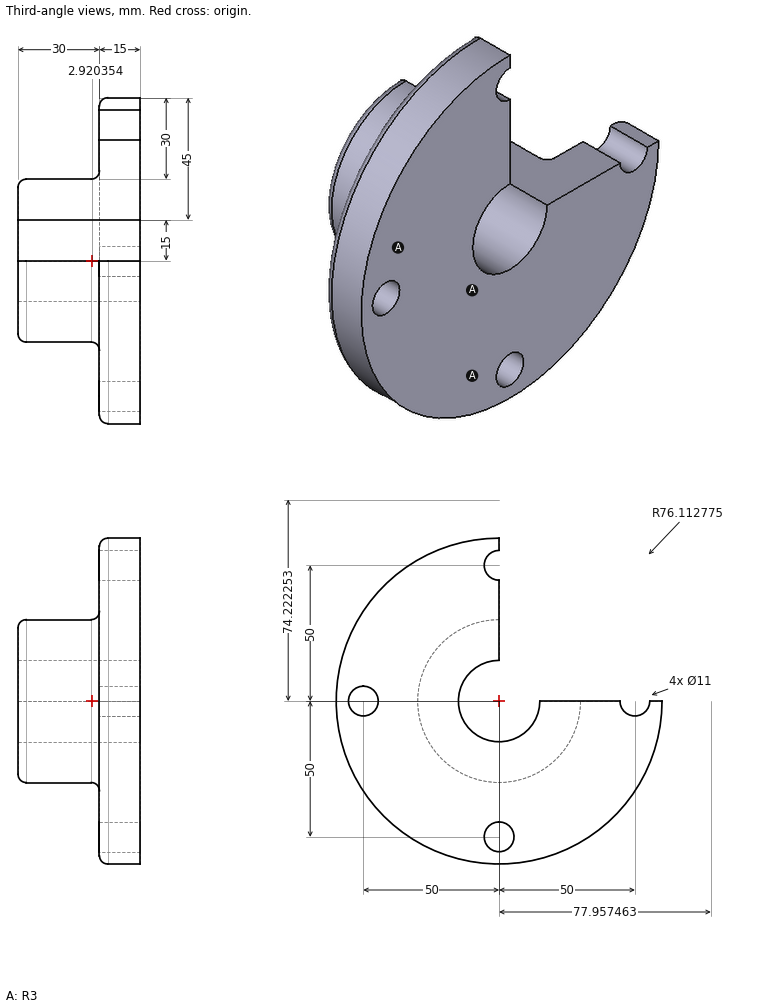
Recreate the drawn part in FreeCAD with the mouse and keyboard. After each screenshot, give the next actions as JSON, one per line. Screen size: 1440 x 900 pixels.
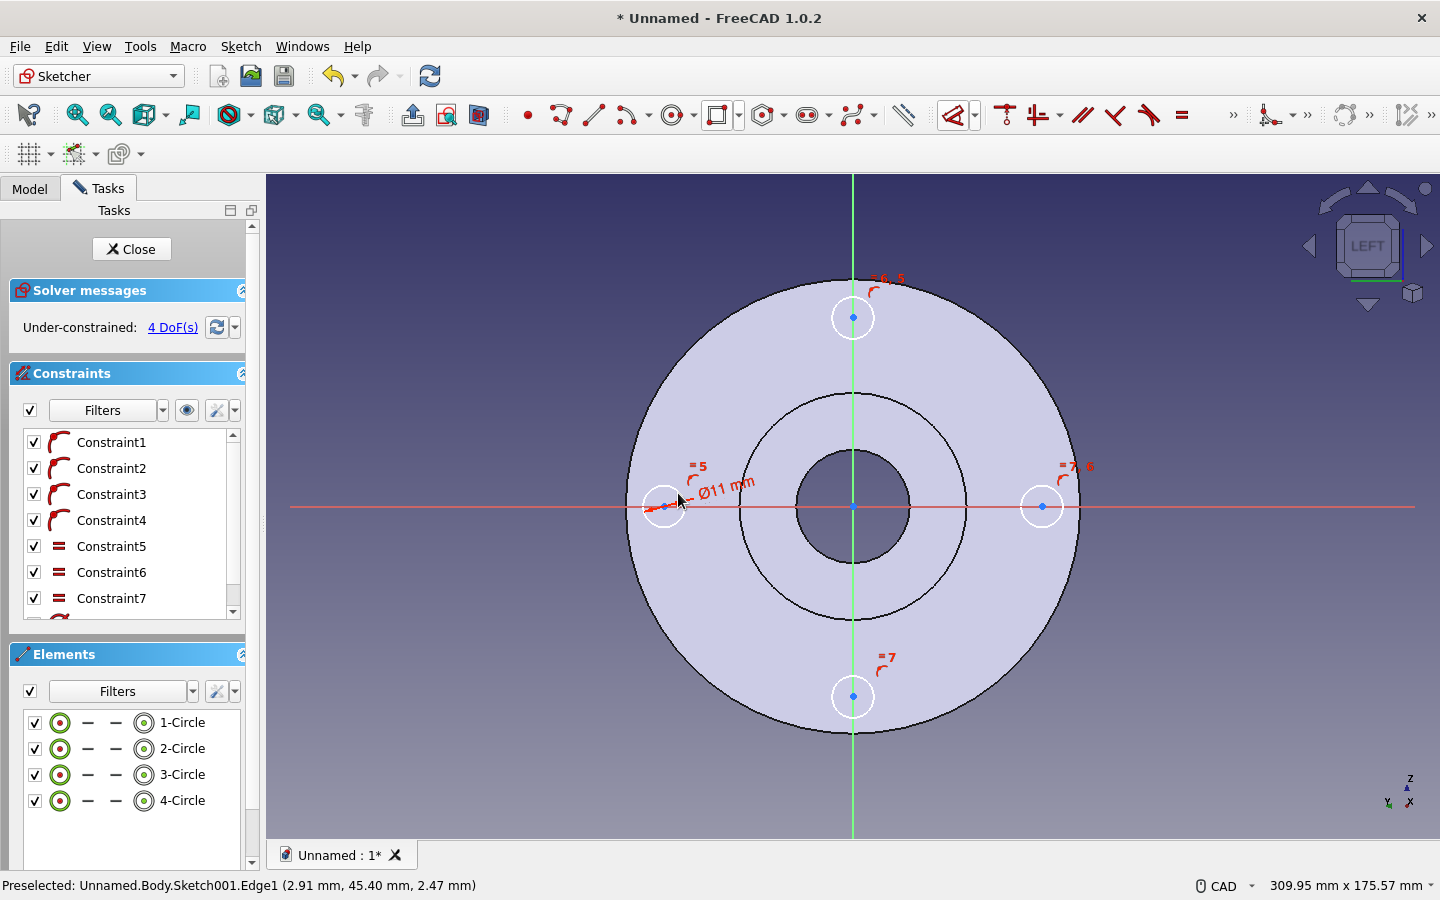
{"action": "left_click", "coordinate": [664, 506]}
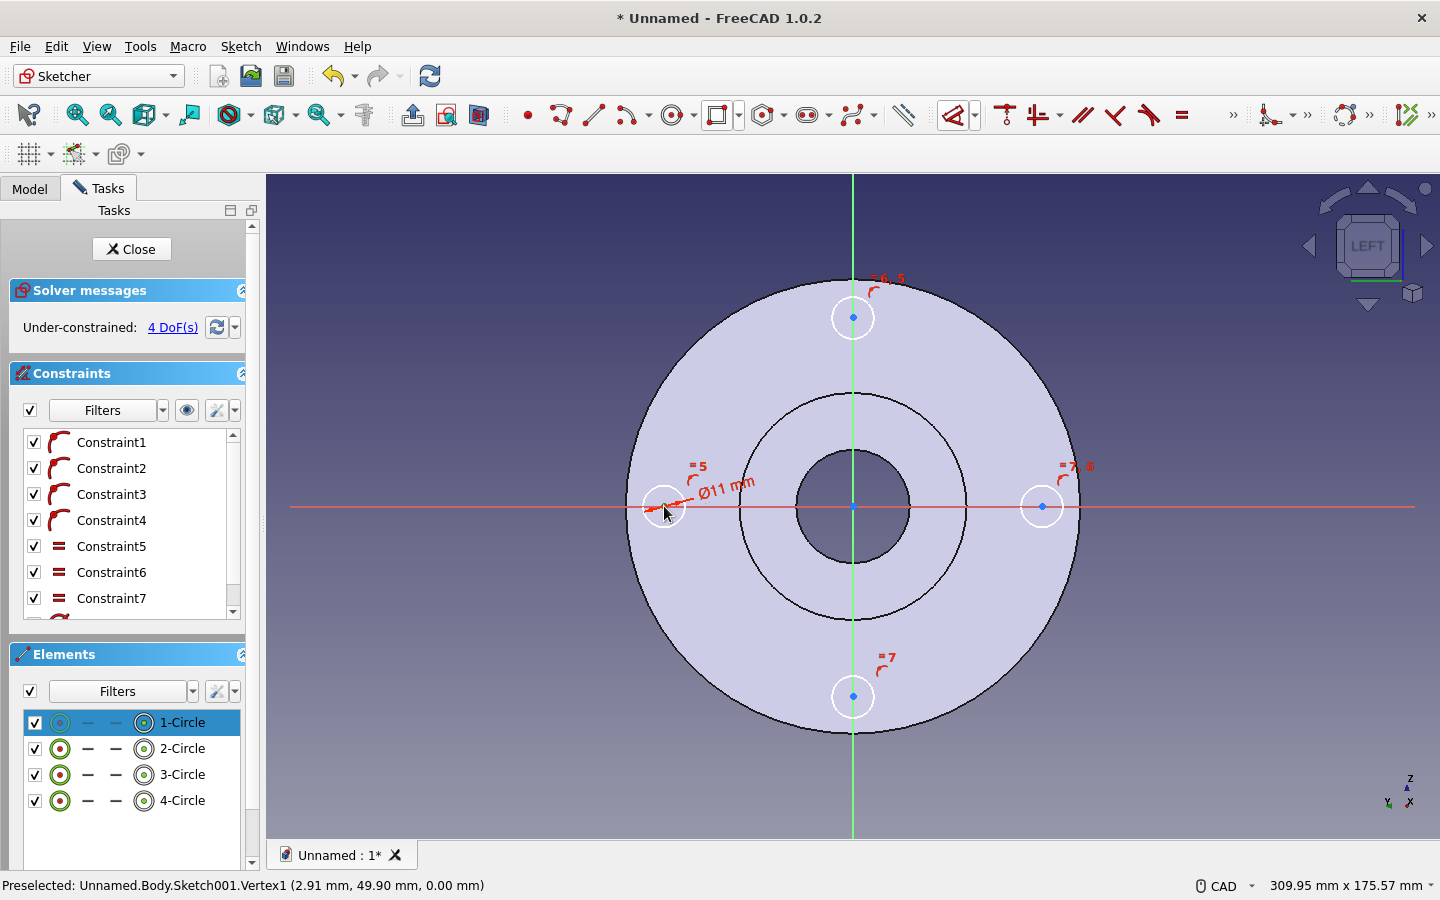
{"action": "left_click", "coordinate": [974, 116]}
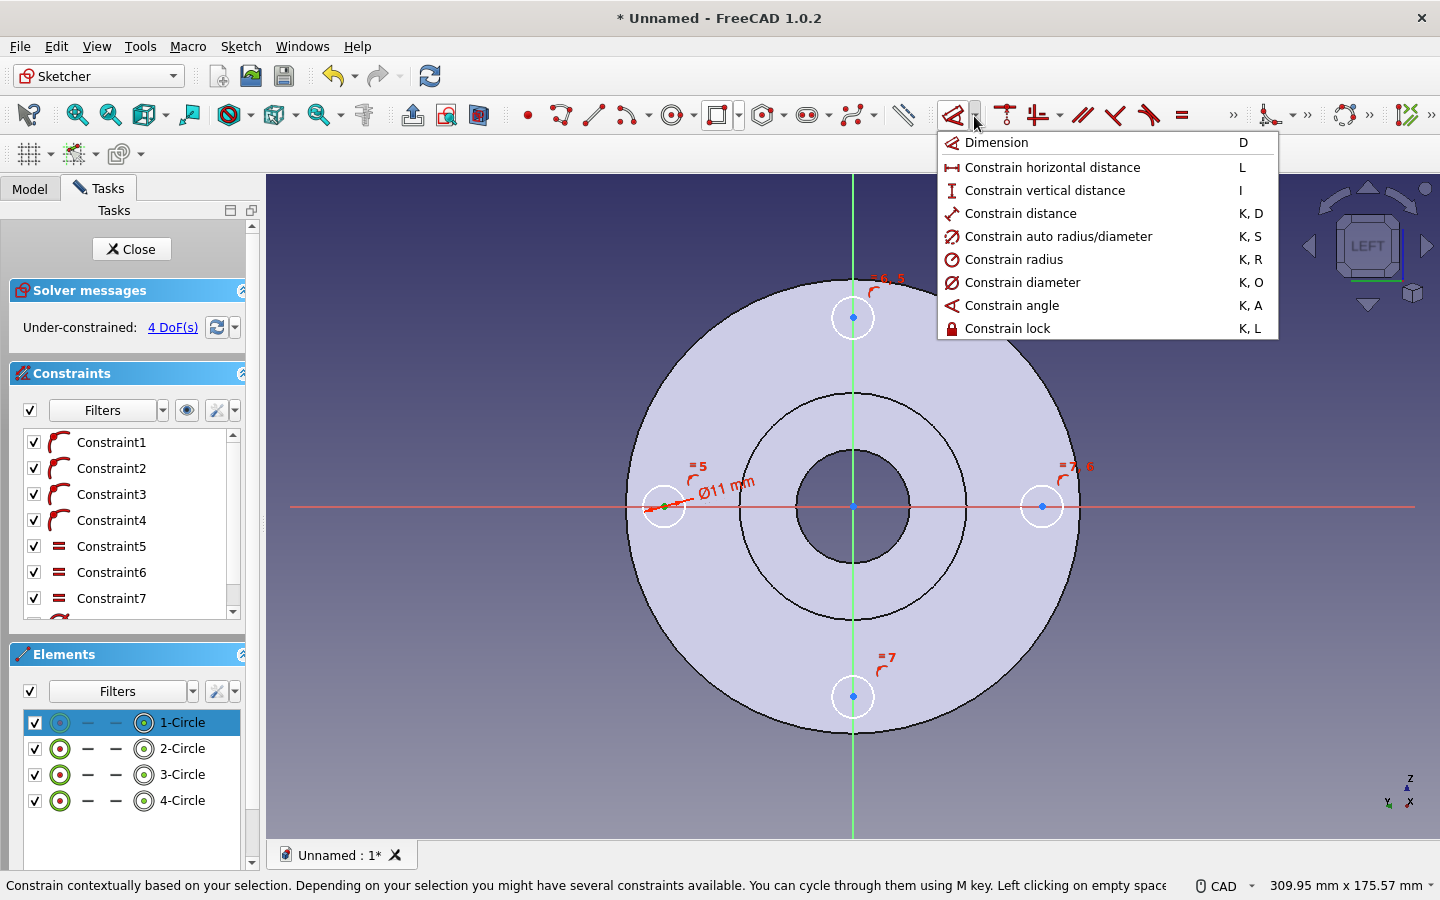
{"action": "left_click", "coordinate": [1108, 168]}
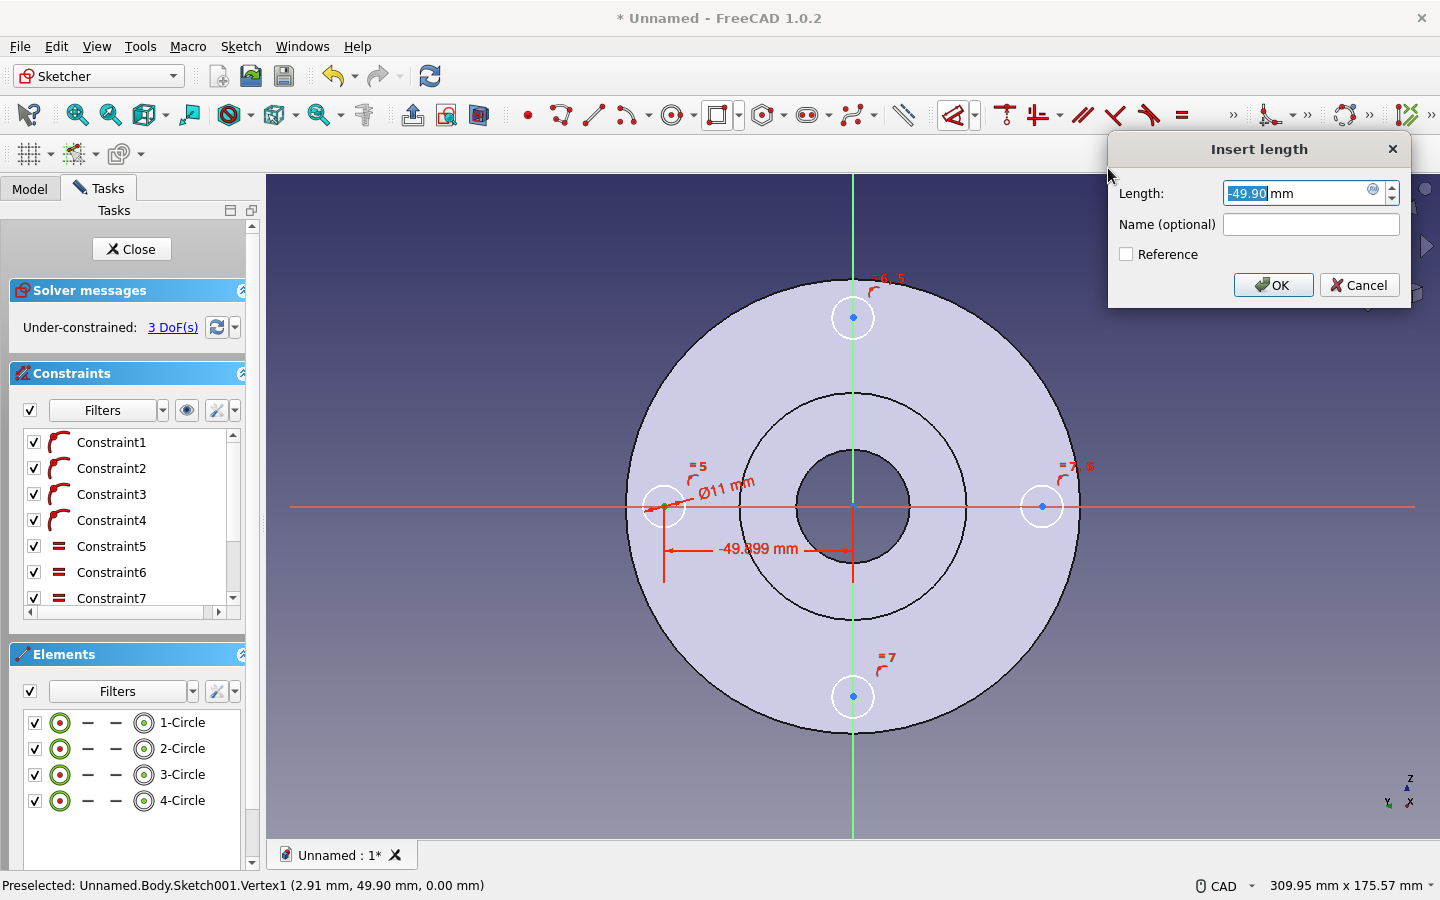
{"action": "type", "text": "-50"}
{"action": "key", "text": "Return"}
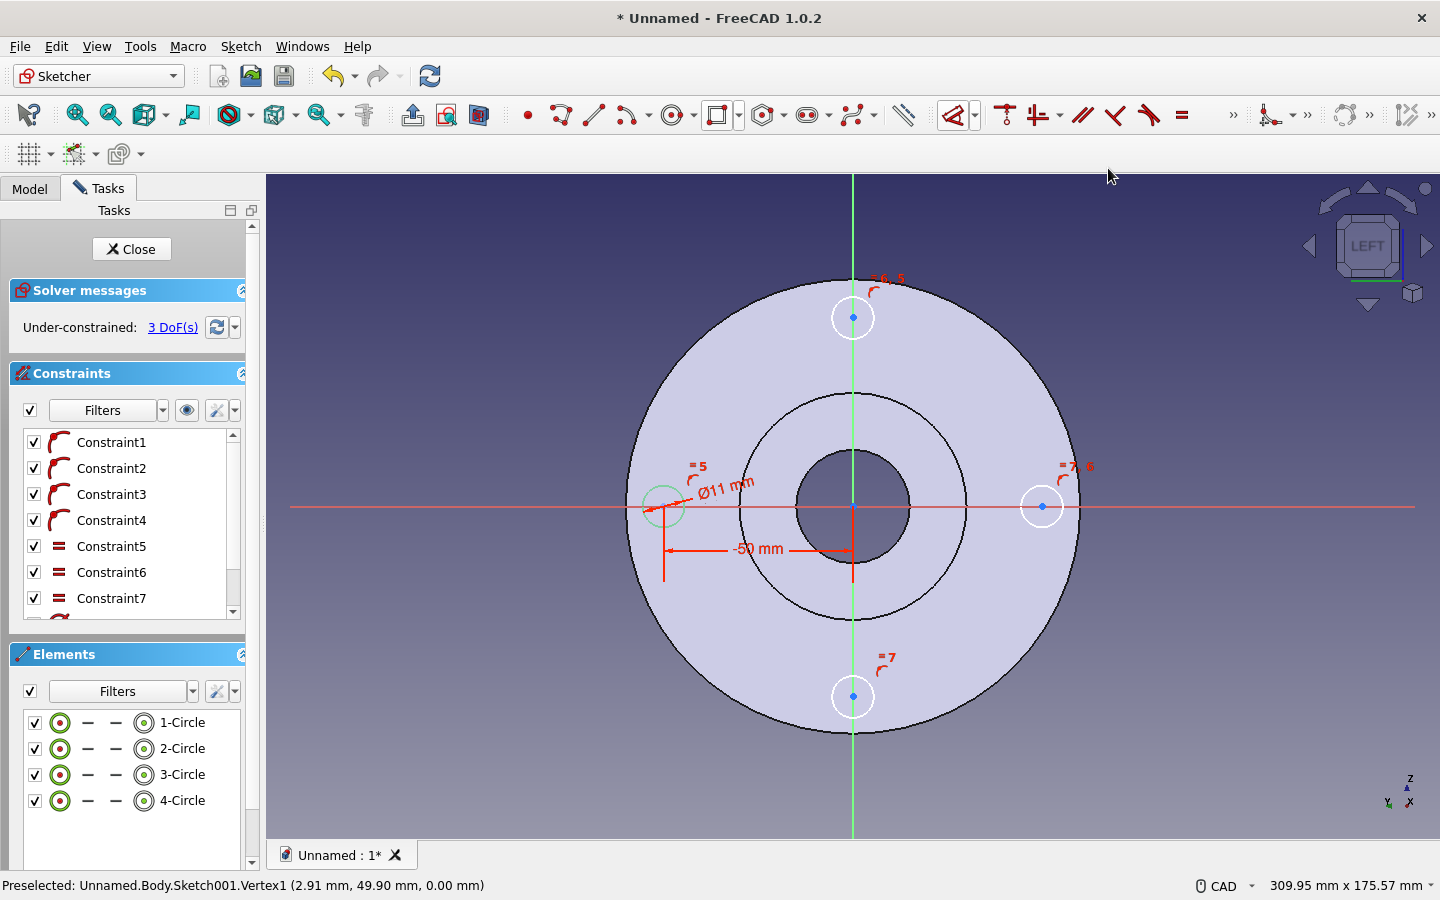
{"action": "left_click", "coordinate": [853, 318]}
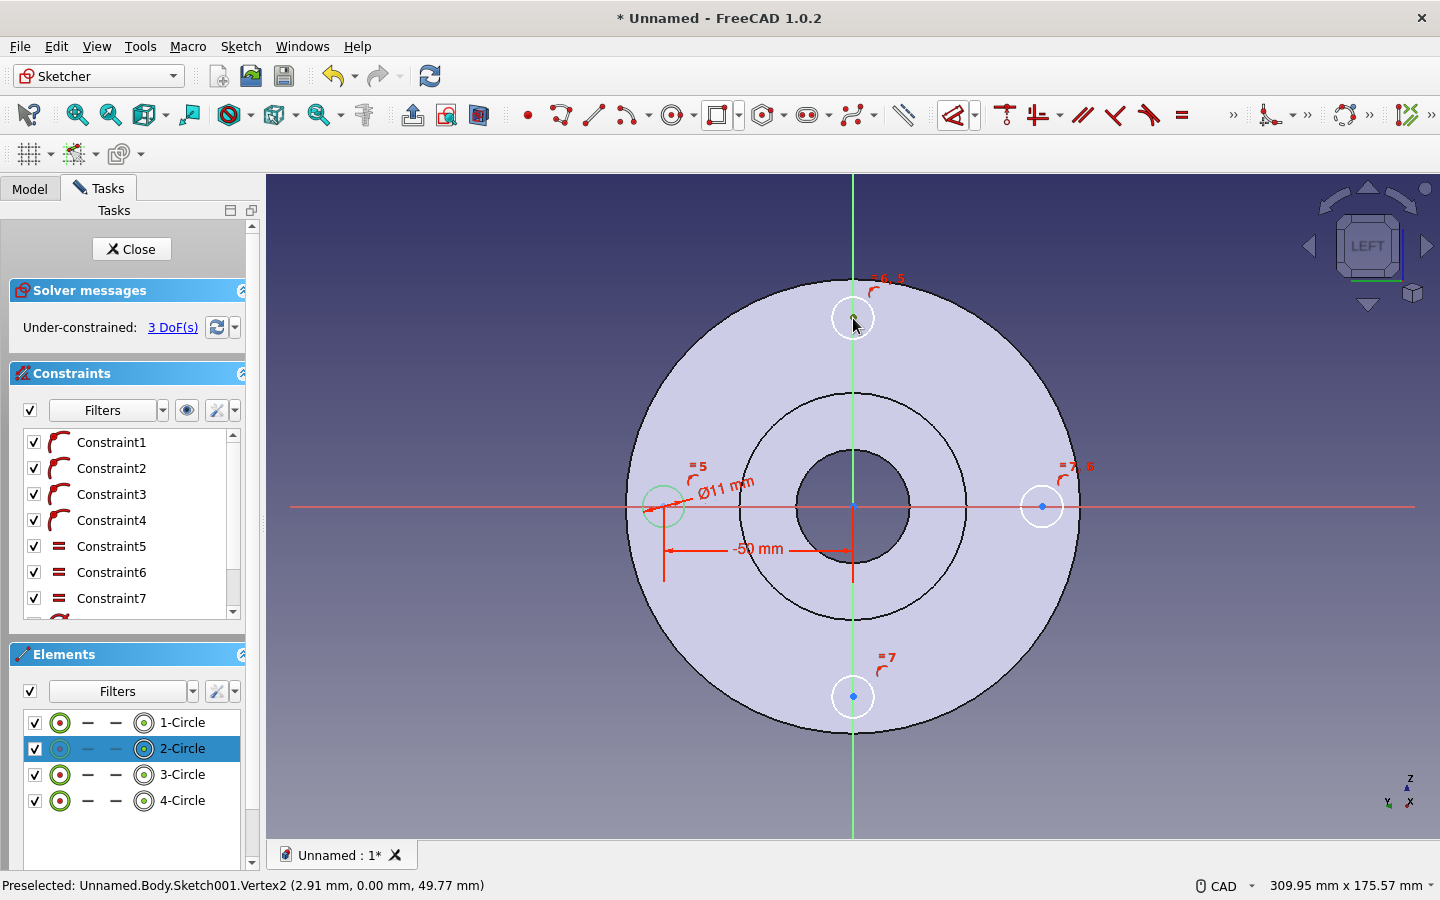
{"action": "left_click", "coordinate": [974, 116]}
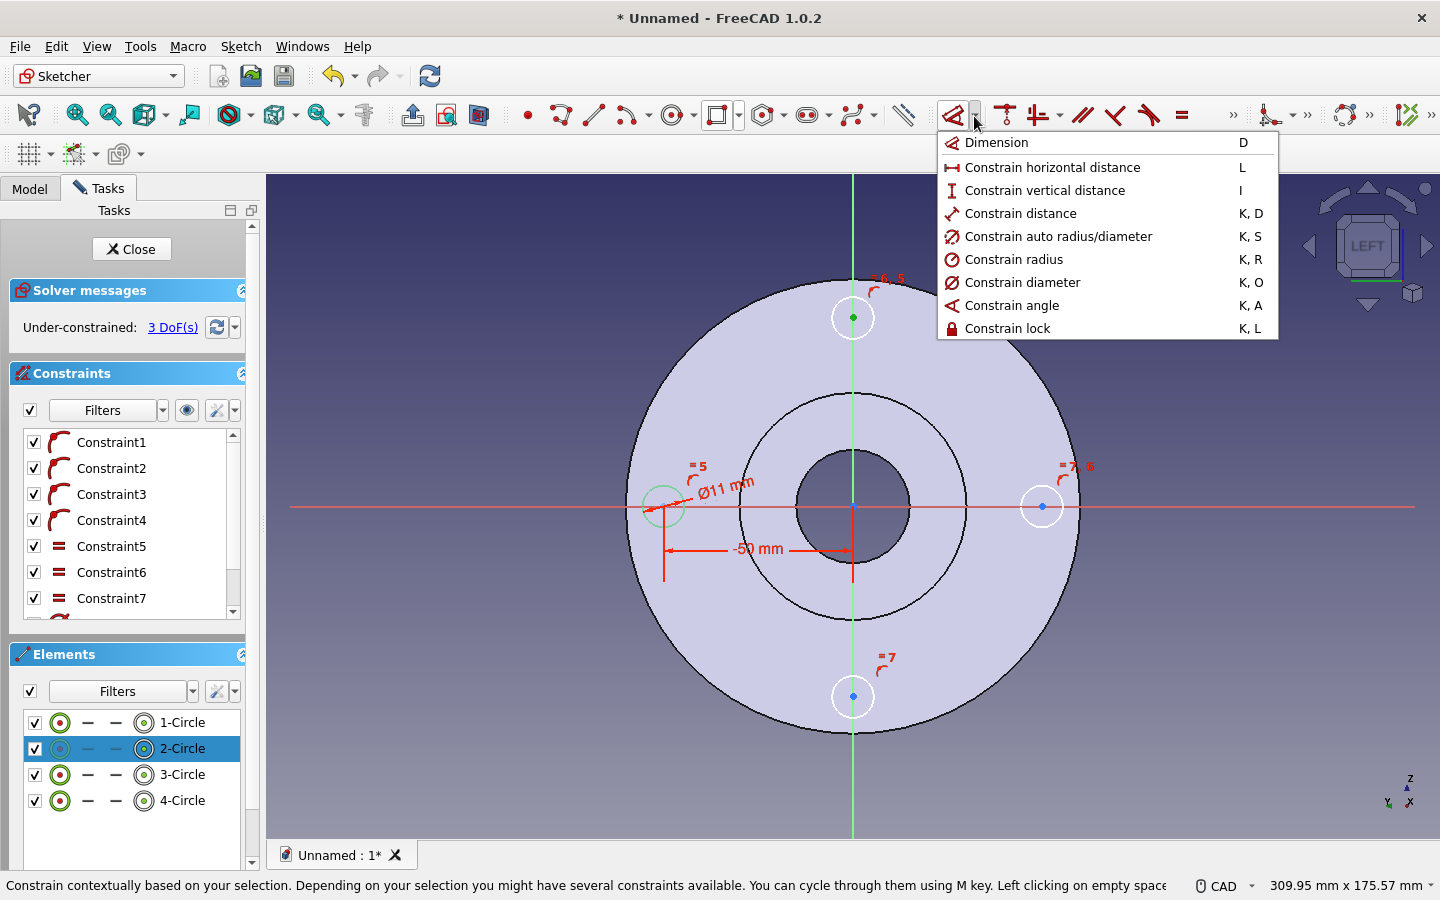
{"action": "left_click", "coordinate": [1108, 190]}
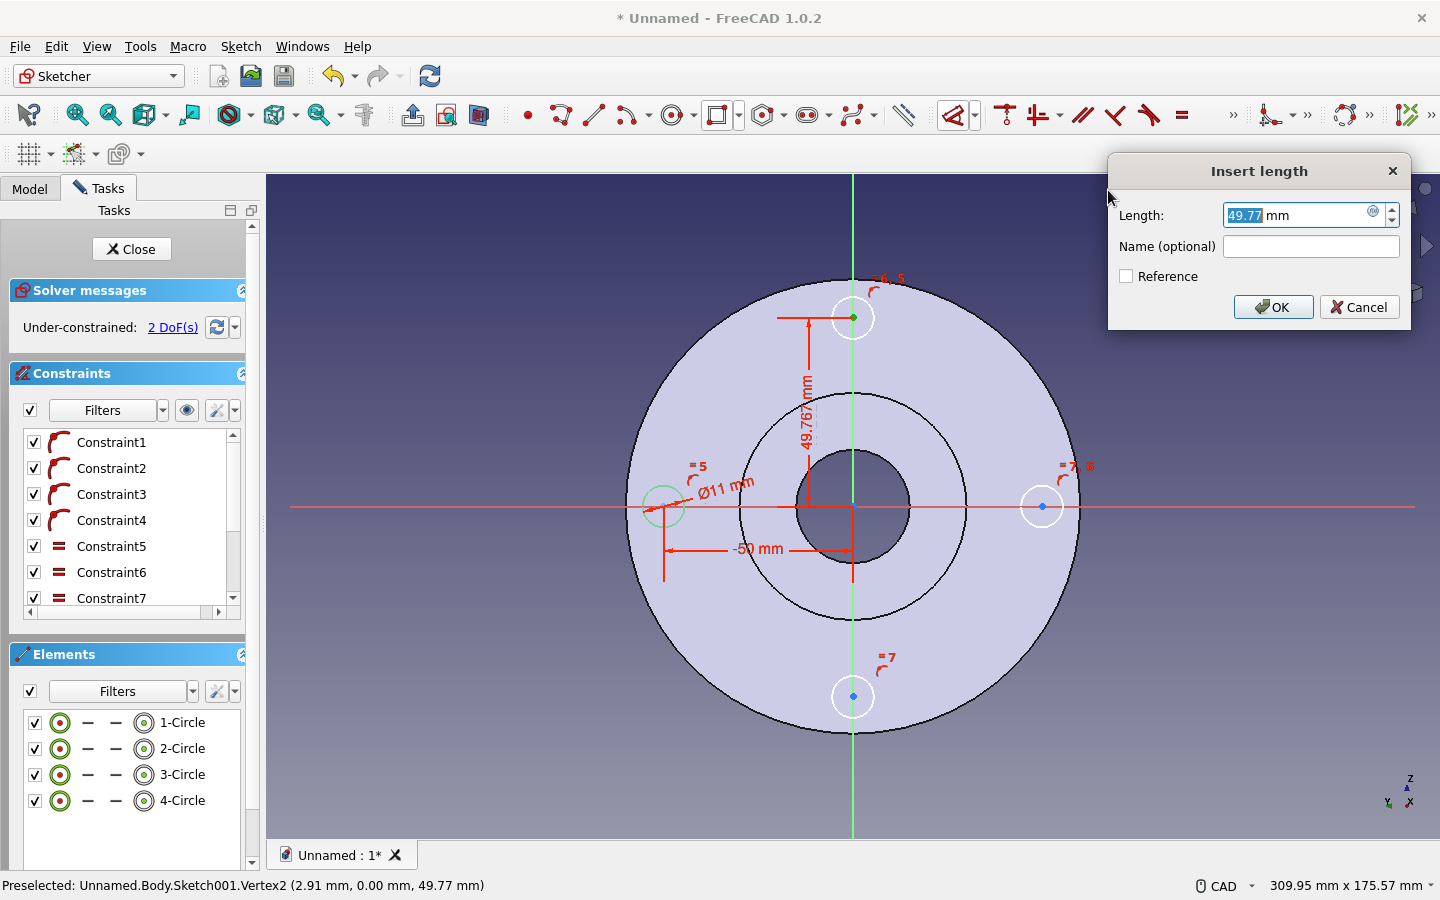
{"action": "type", "text": "50"}
{"action": "key", "text": "Return"}